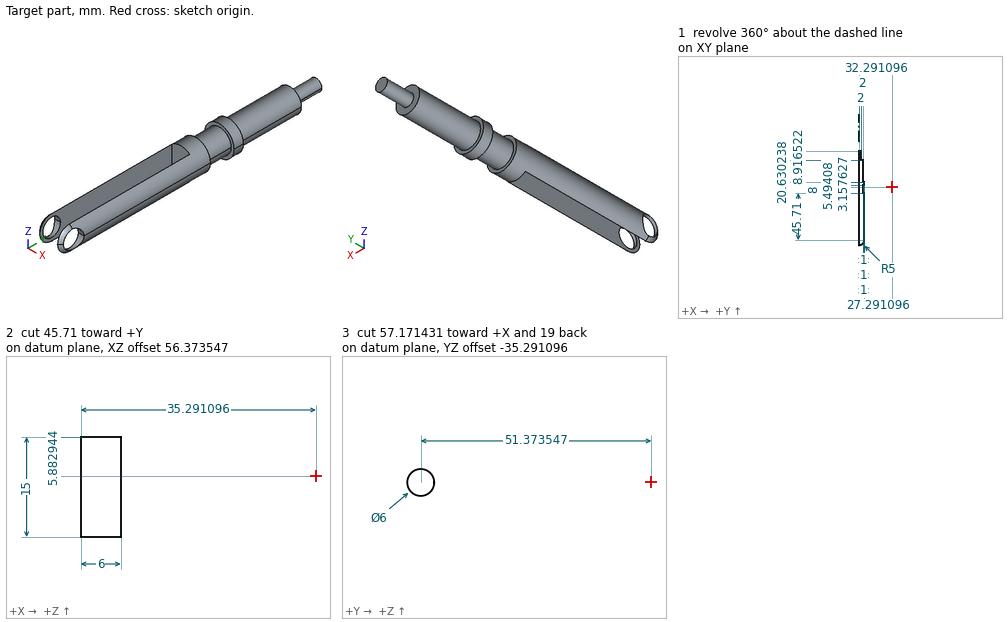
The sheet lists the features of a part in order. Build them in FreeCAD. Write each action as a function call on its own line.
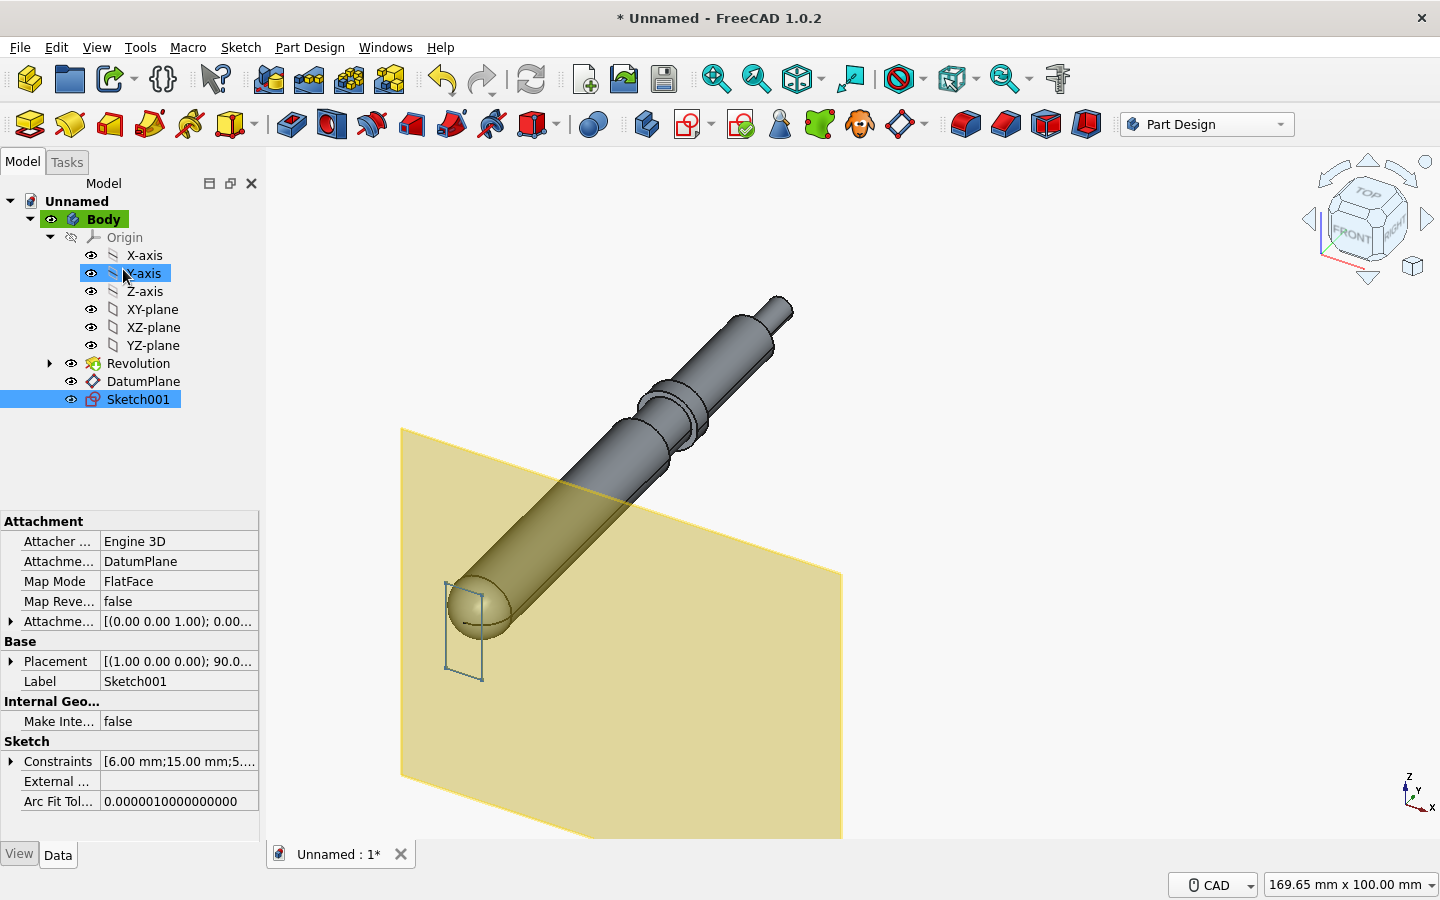
click(292, 124)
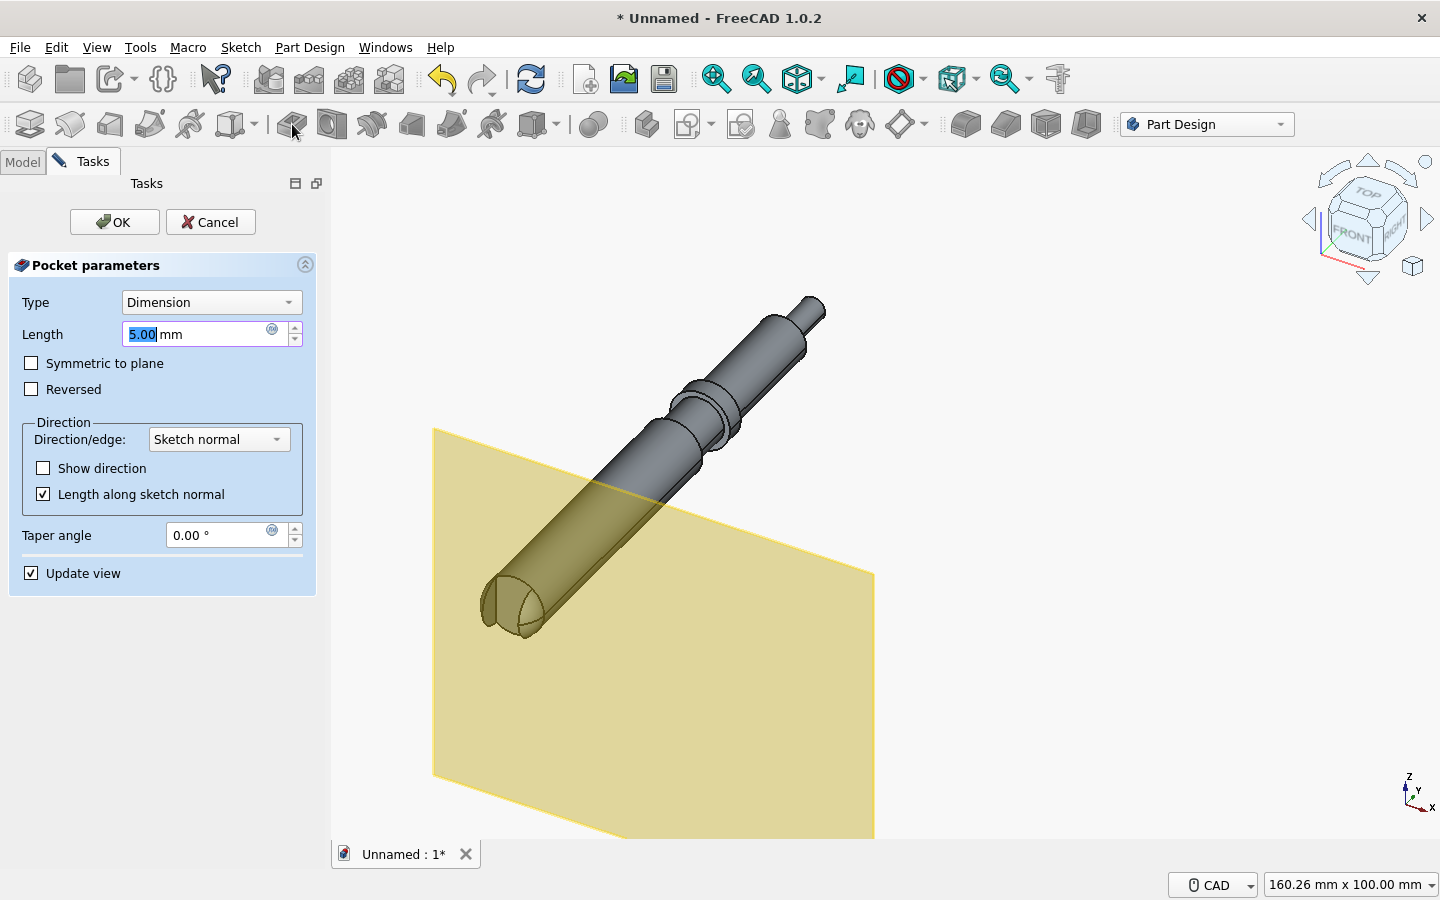
text(45.71)
key(Tab)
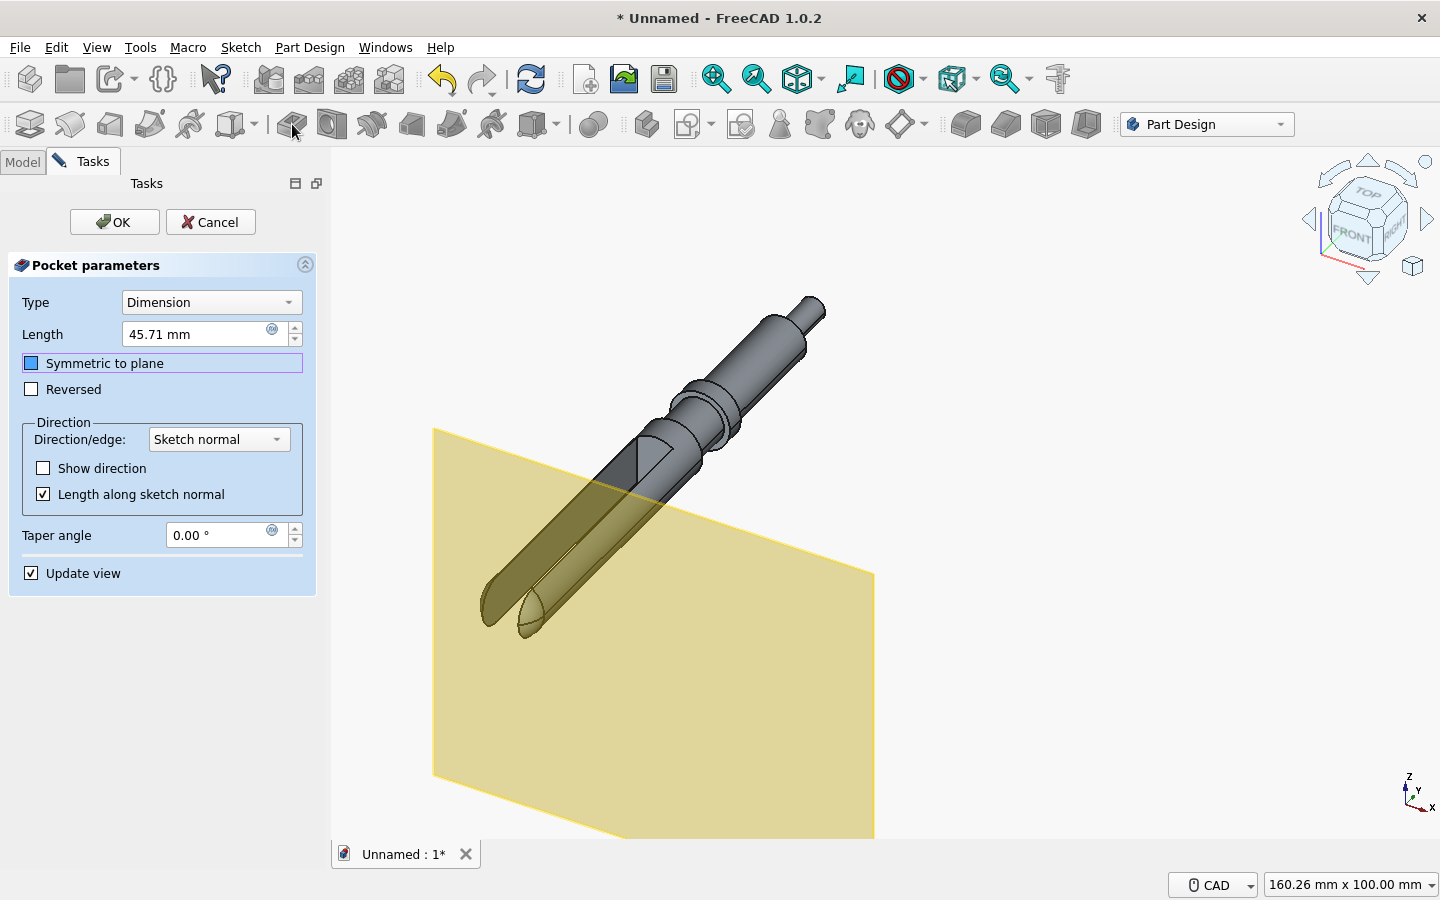
click(115, 222)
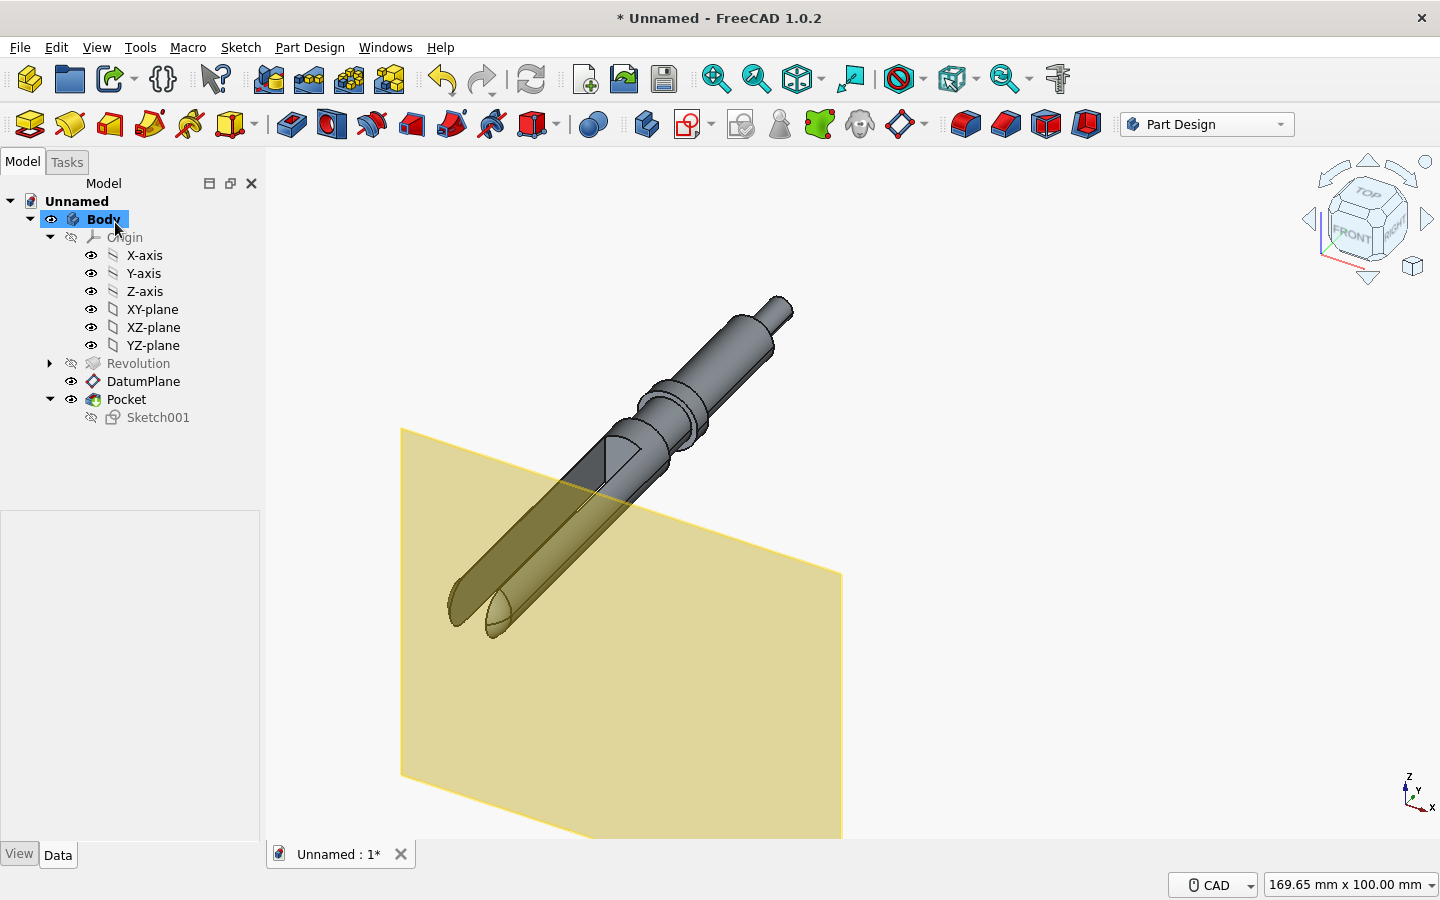
click(116, 381)
key(space)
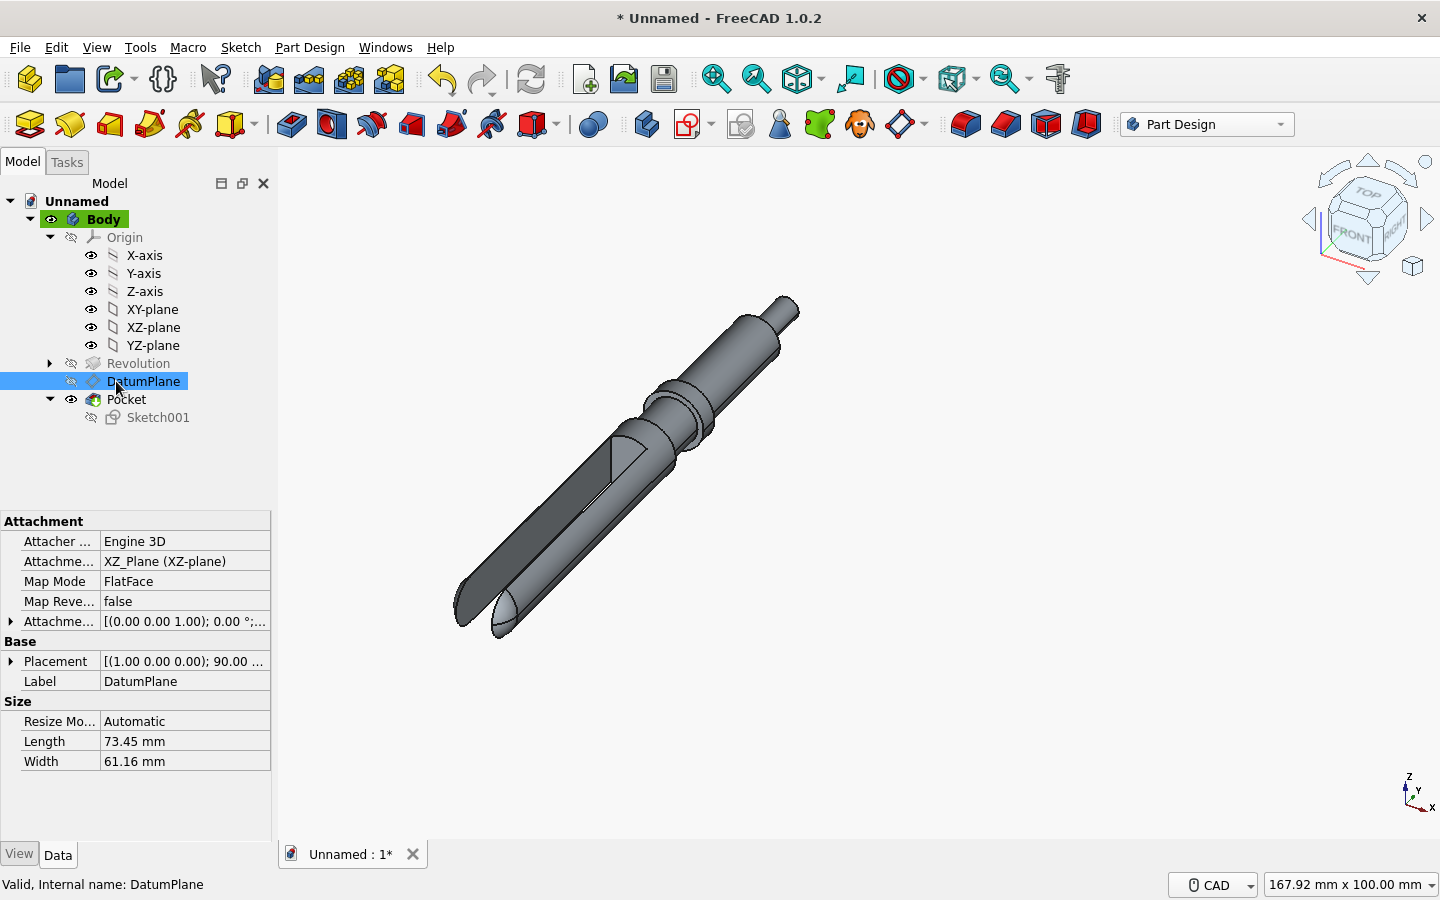
click(136, 345)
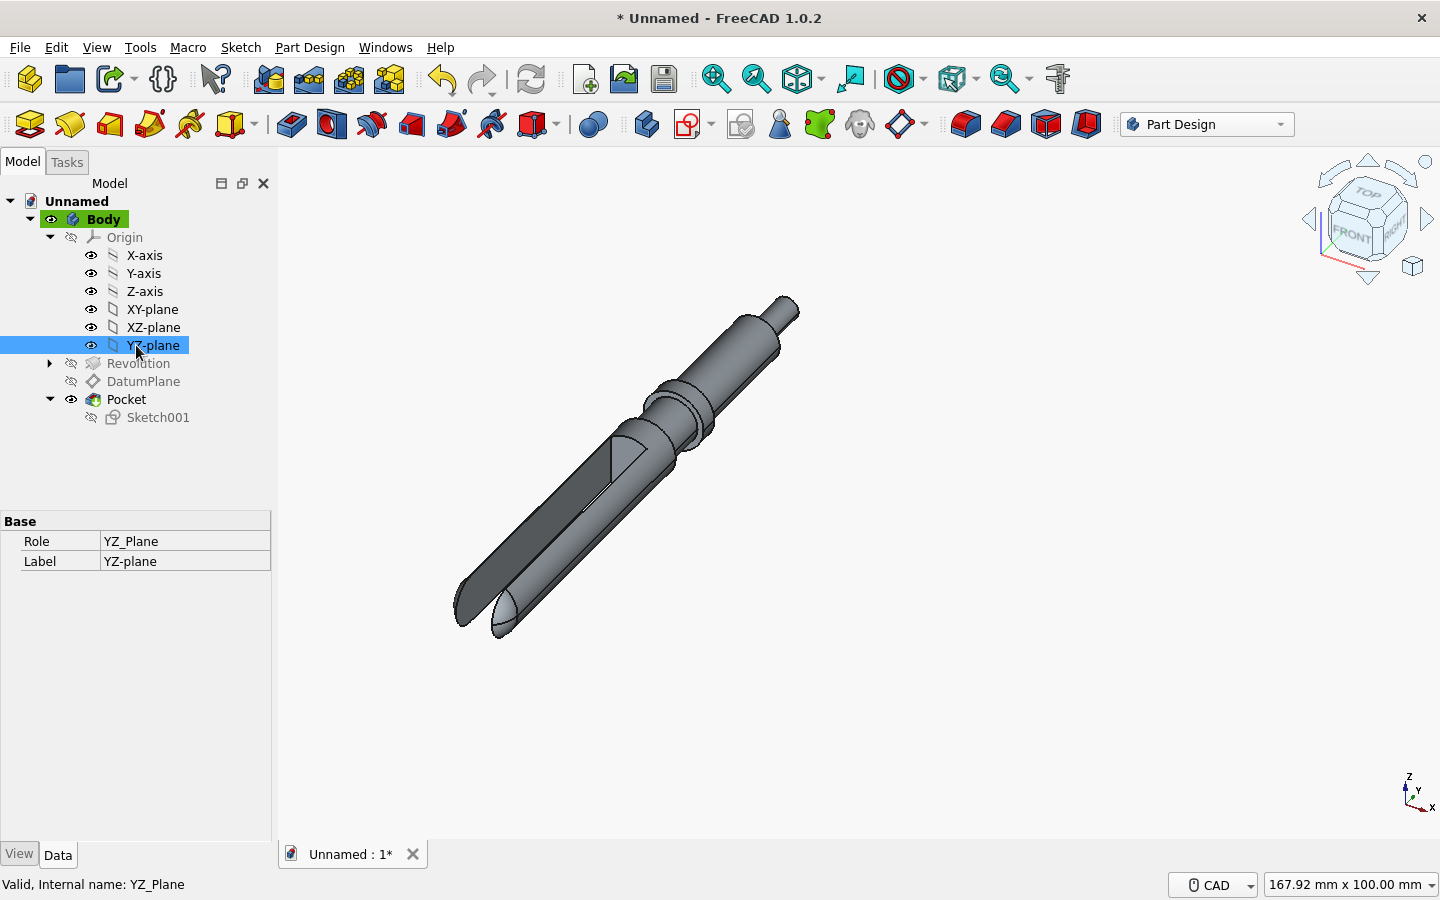
click(900, 124)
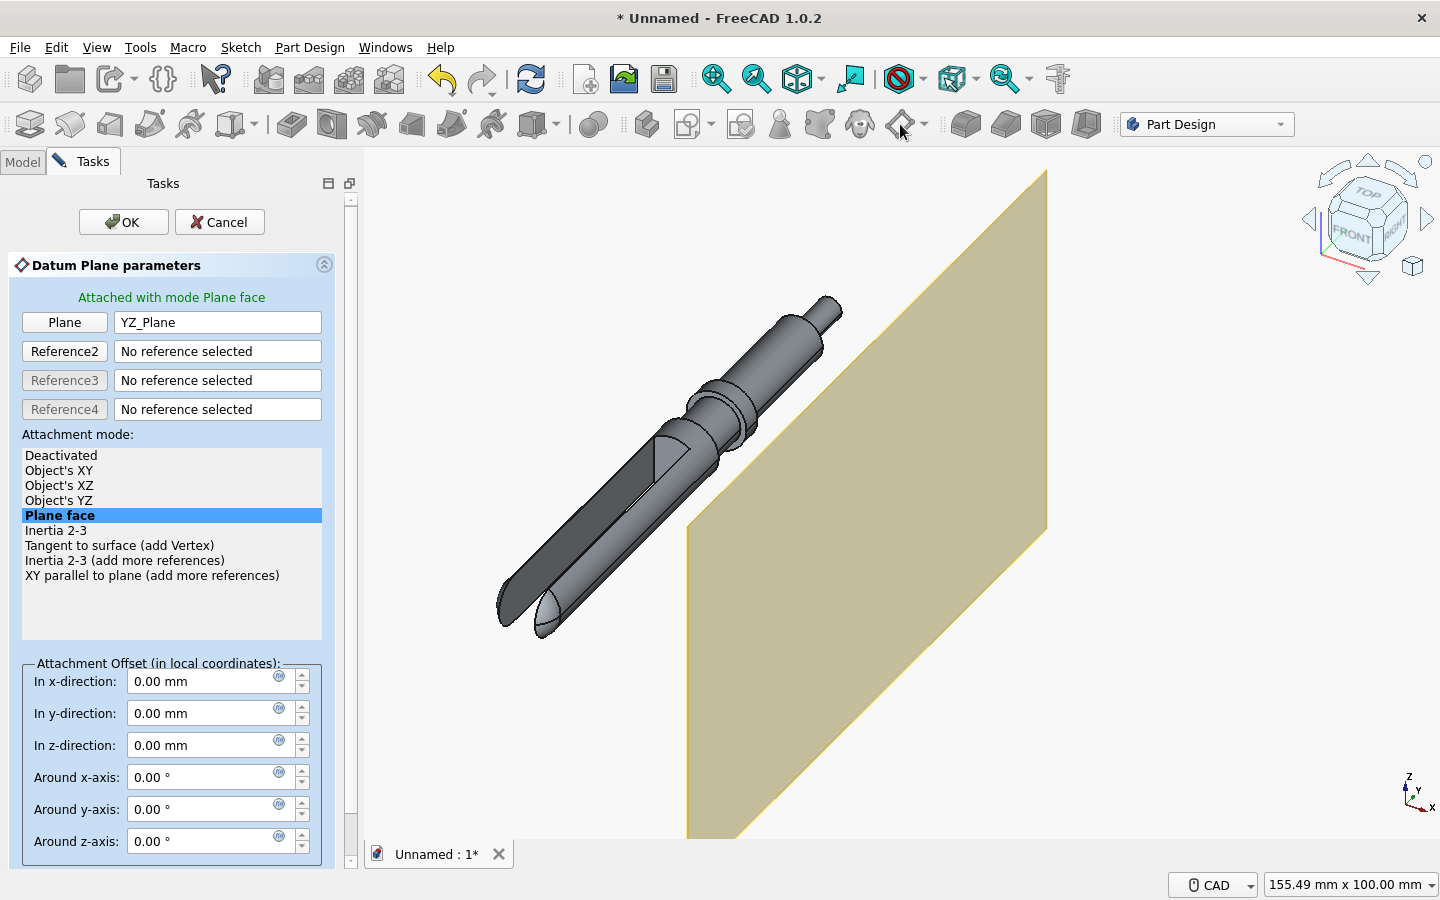
triple_click(210, 745)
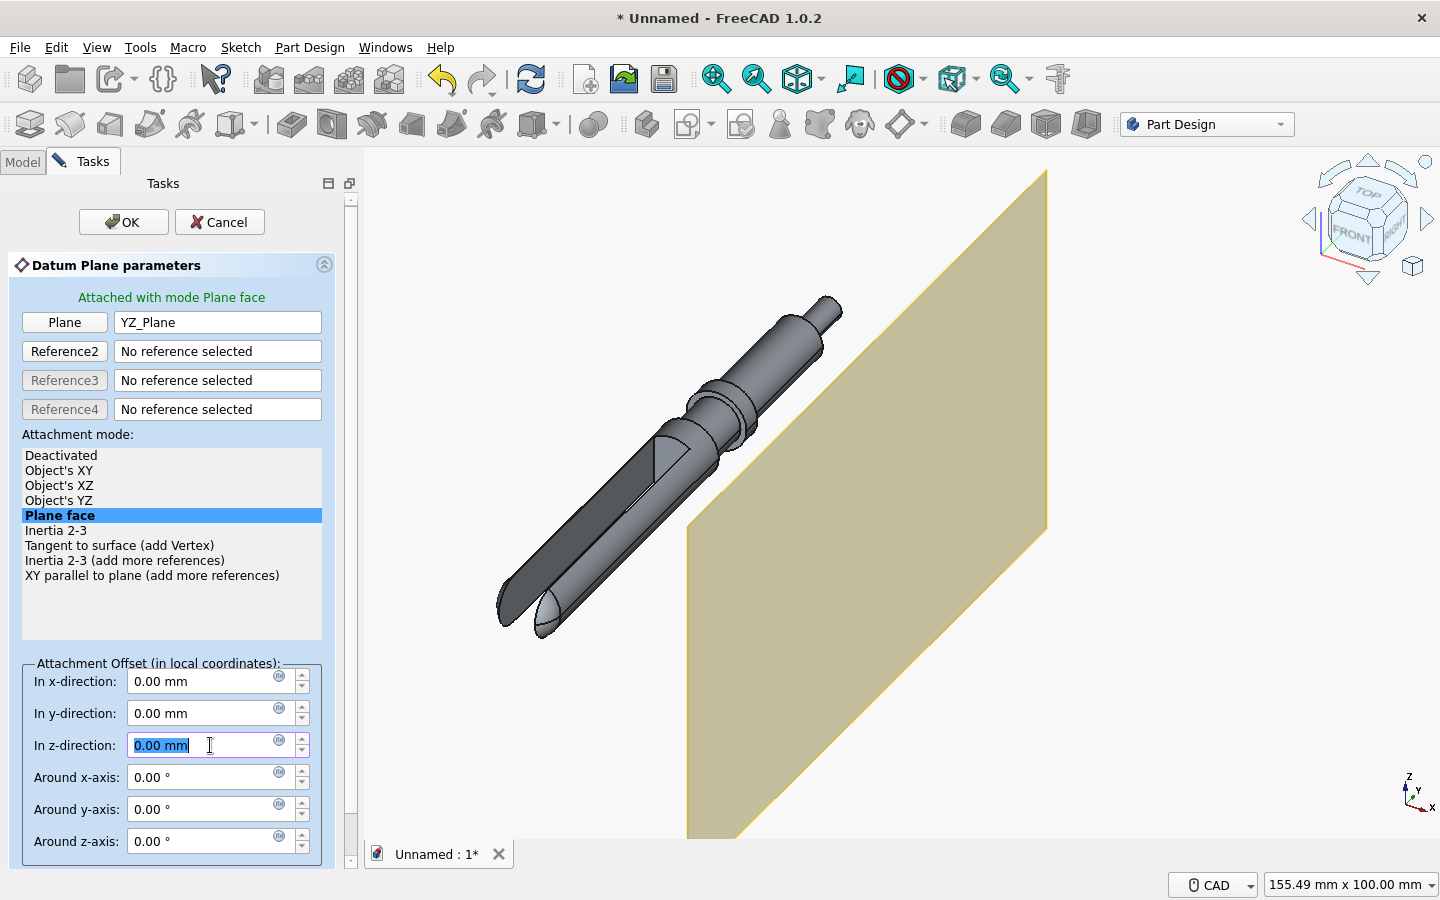
text(-35.291096)
key(Tab)